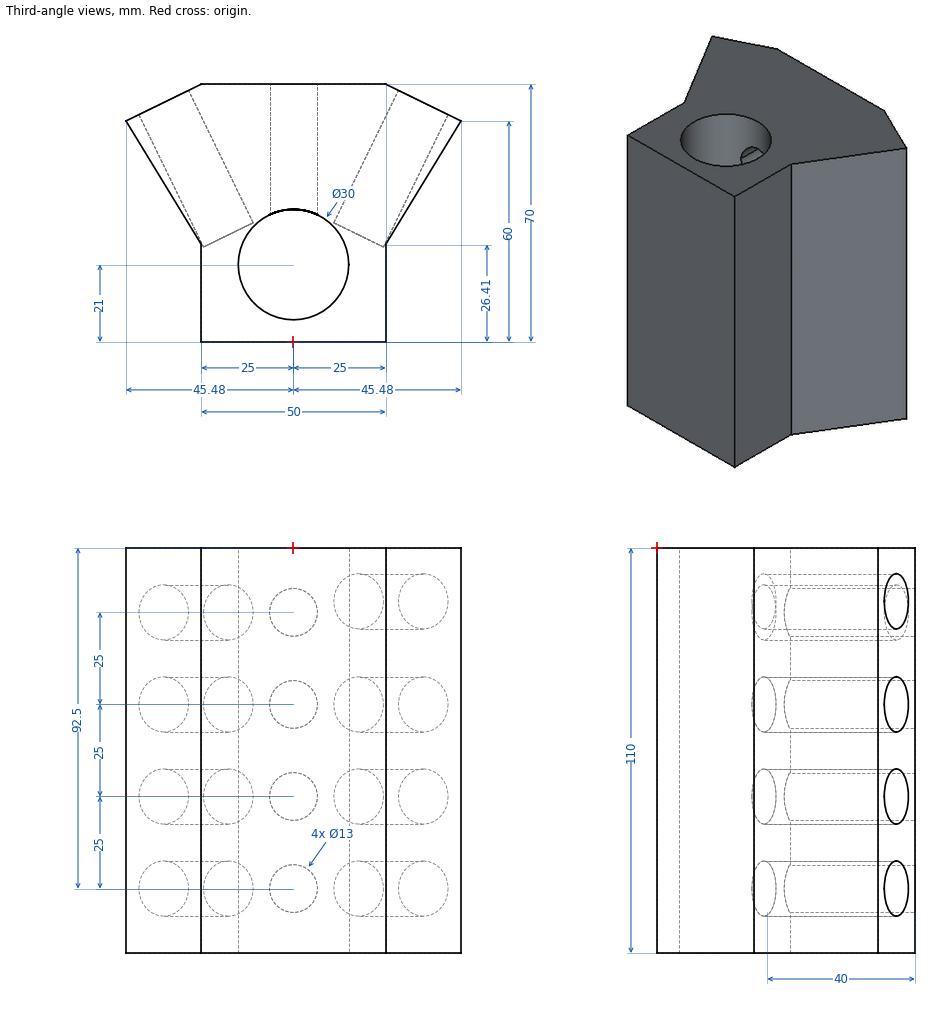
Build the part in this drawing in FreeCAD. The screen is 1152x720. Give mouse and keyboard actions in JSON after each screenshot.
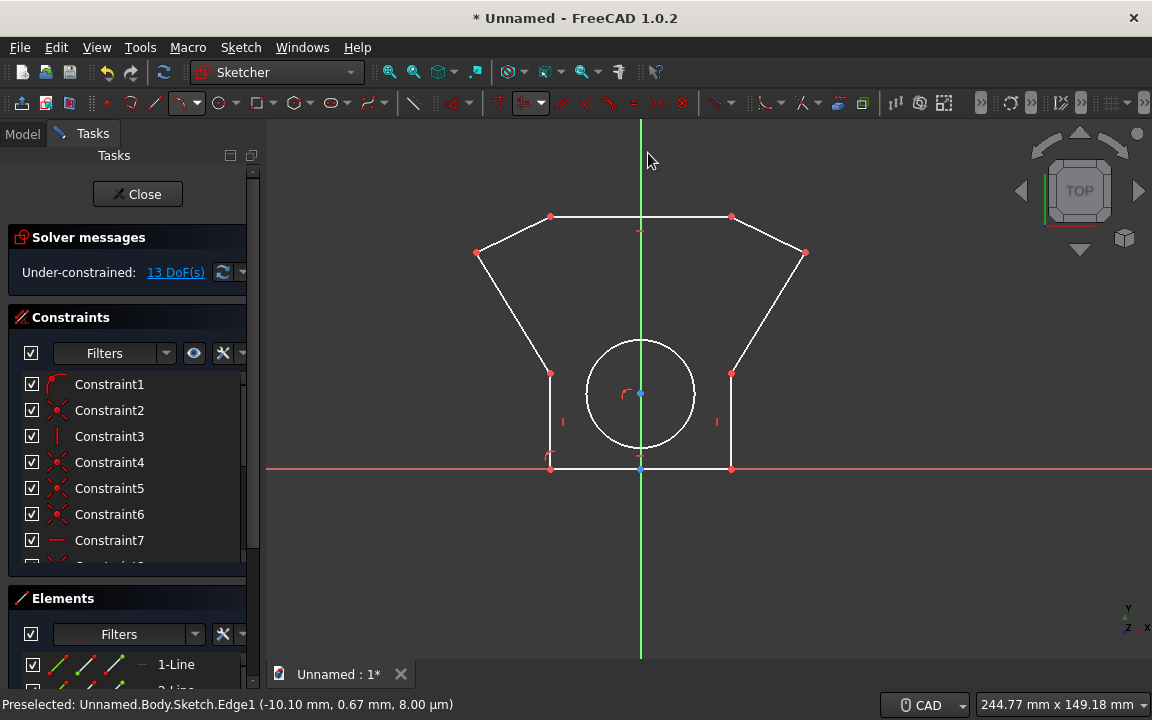
{"action": "left_click", "coordinate": [452, 104]}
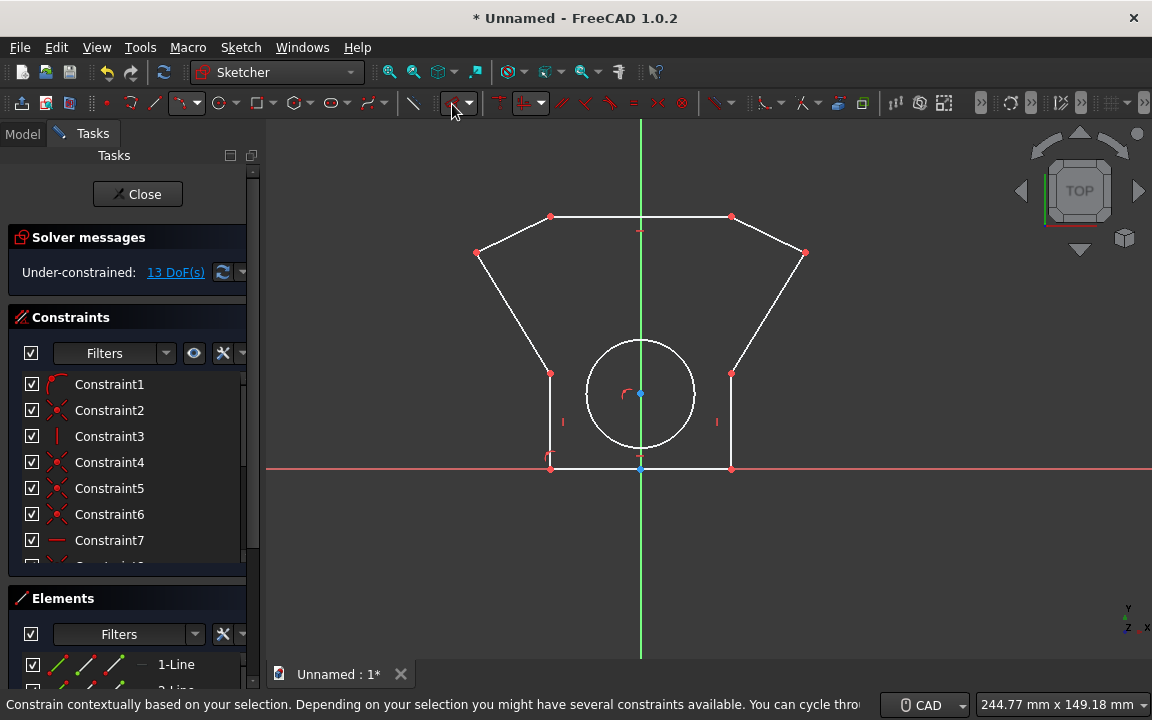
{"action": "left_click", "coordinate": [679, 356]}
{"action": "left_click", "coordinate": [702, 334]}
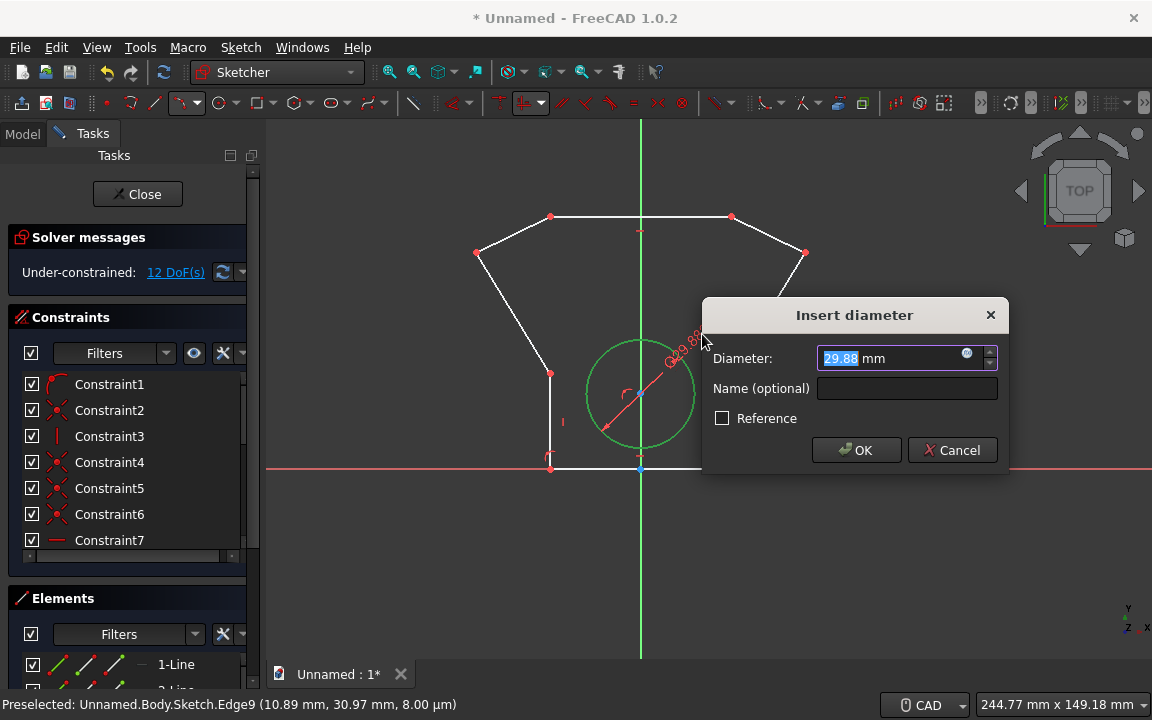
{"action": "type", "text": "30"}
{"action": "key", "text": "Return"}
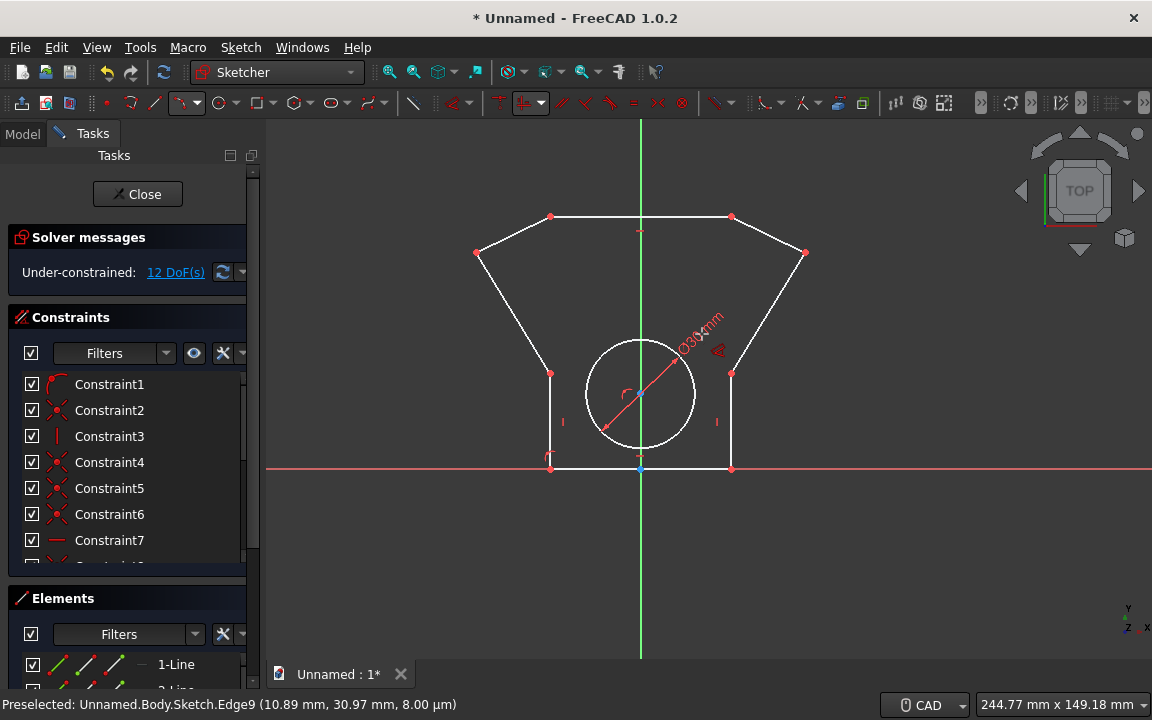
{"action": "left_click", "coordinate": [604, 469]}
{"action": "left_click", "coordinate": [599, 503]}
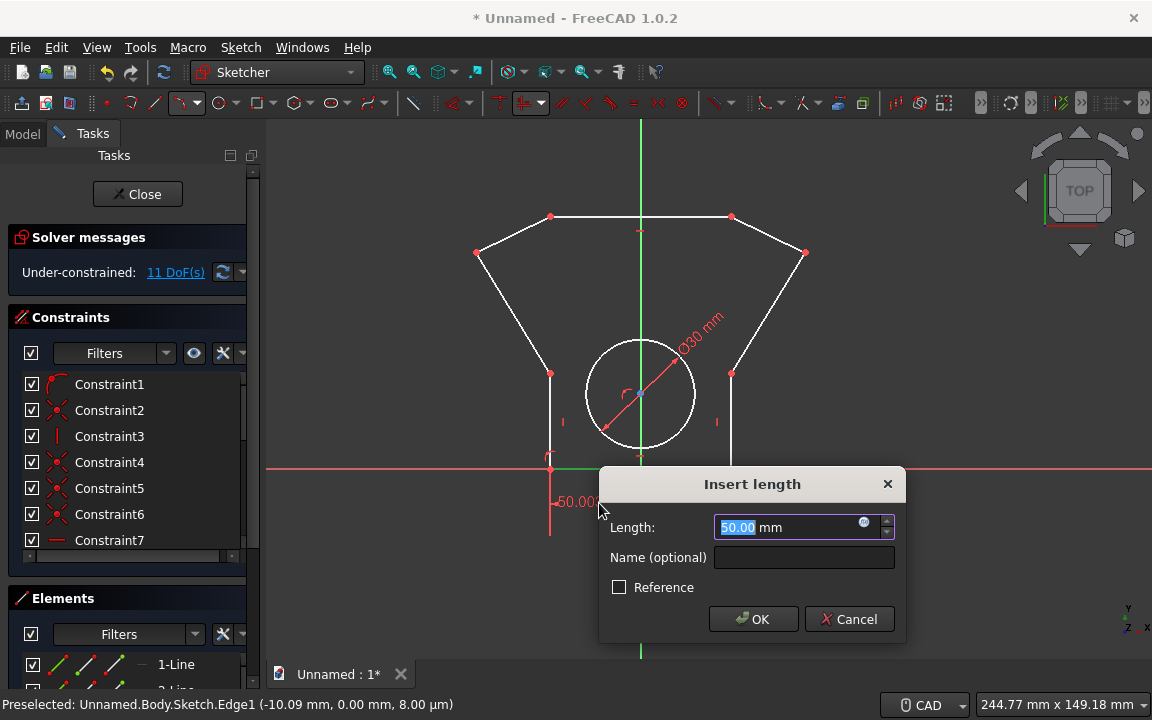
{"action": "type", "text": "50"}
{"action": "key", "text": "Return"}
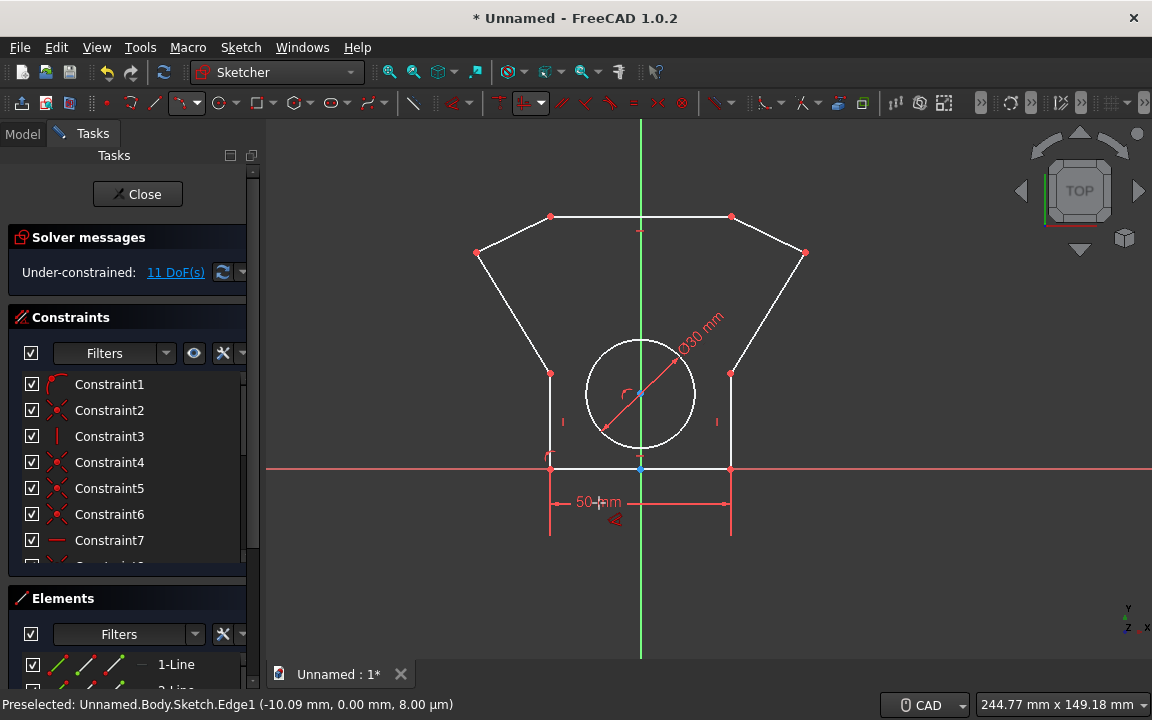
{"action": "left_click", "coordinate": [677, 217]}
{"action": "left_click", "coordinate": [599, 183]}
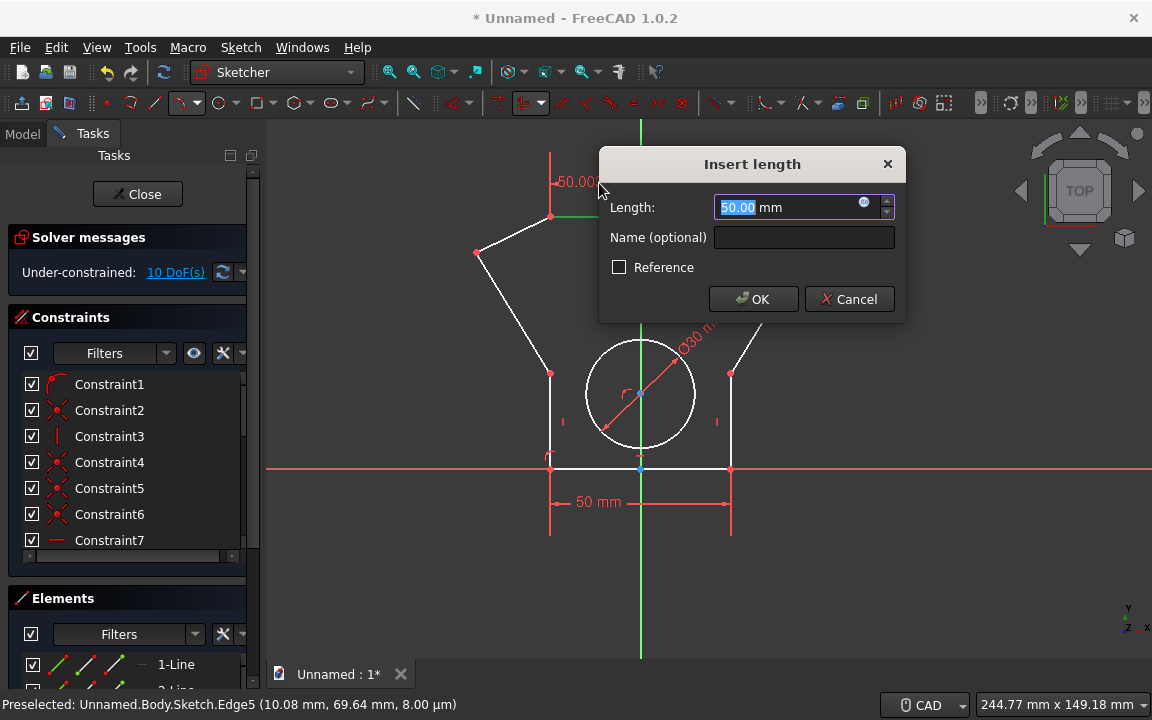
{"action": "type", "text": "50"}
{"action": "key", "text": "Return"}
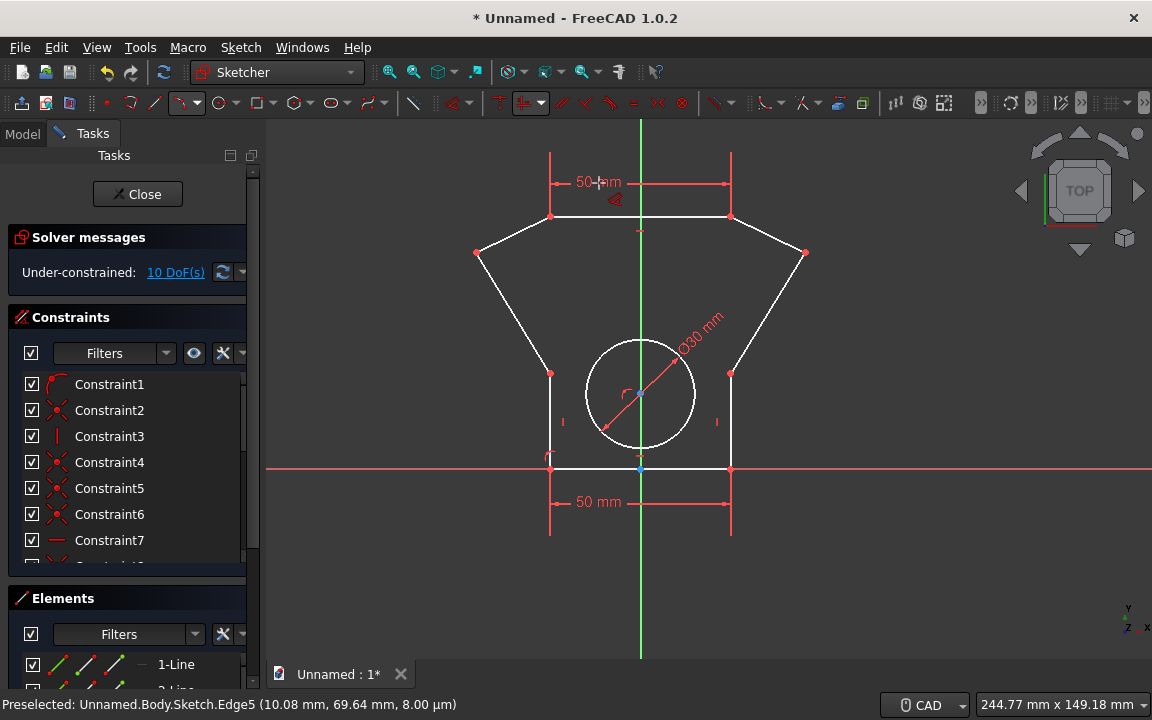
{"action": "left_click", "coordinate": [641, 394]}
{"action": "left_click", "coordinate": [675, 414]}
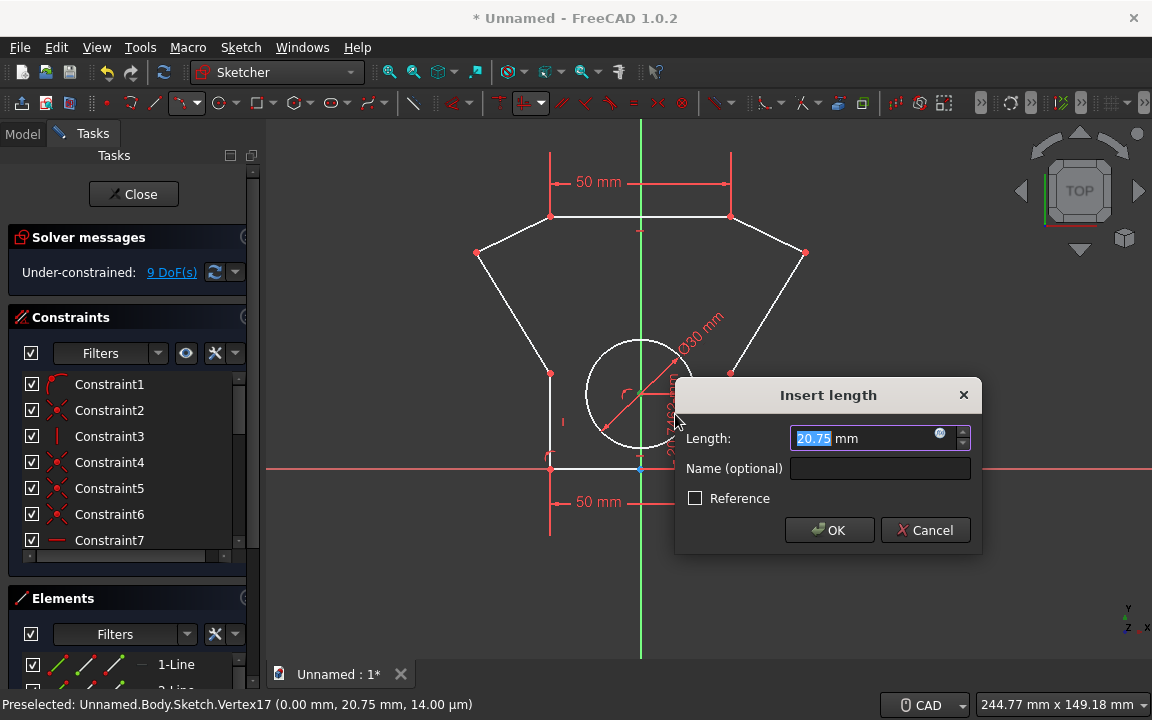
{"action": "type", "text": "21"}
{"action": "key", "text": "Return"}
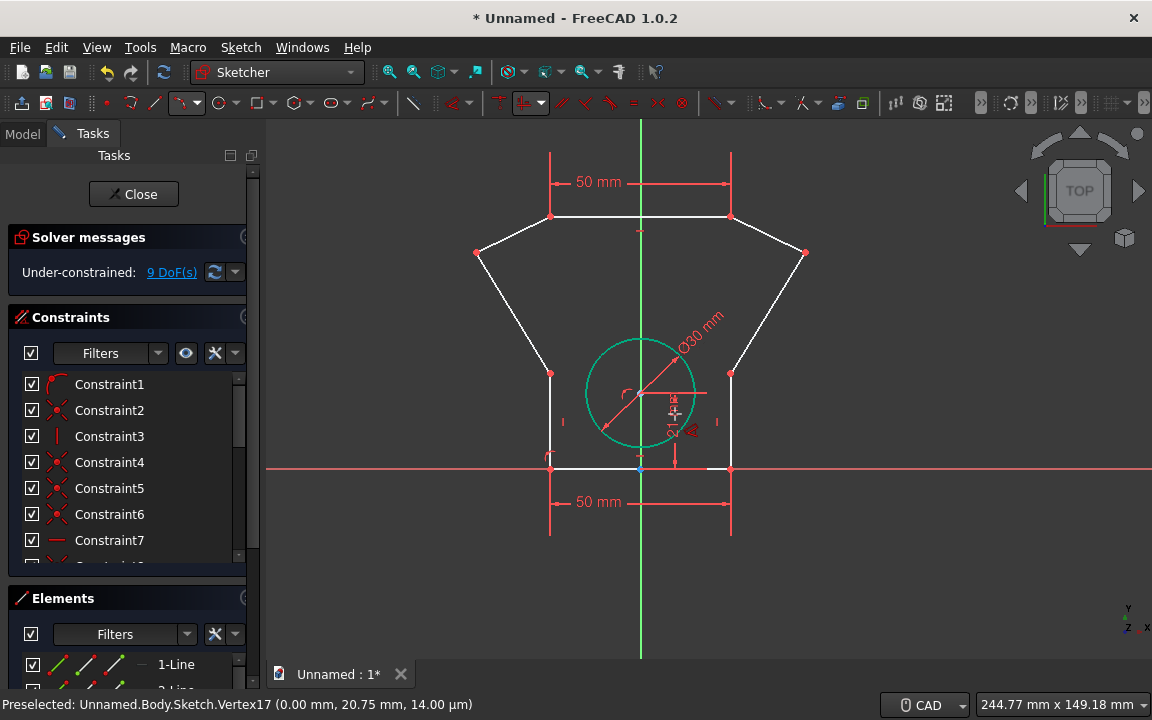
{"action": "left_click", "coordinate": [550, 469]}
{"action": "left_click", "coordinate": [574, 435]}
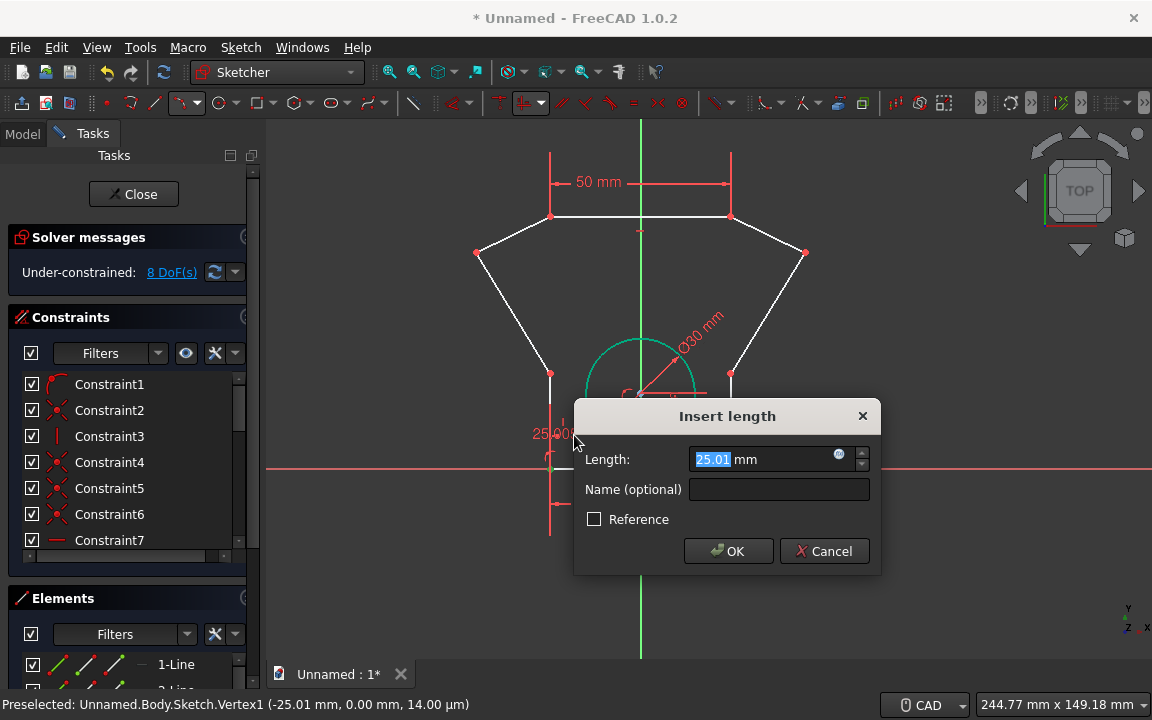
{"action": "type", "text": "25"}
{"action": "key", "text": "Return"}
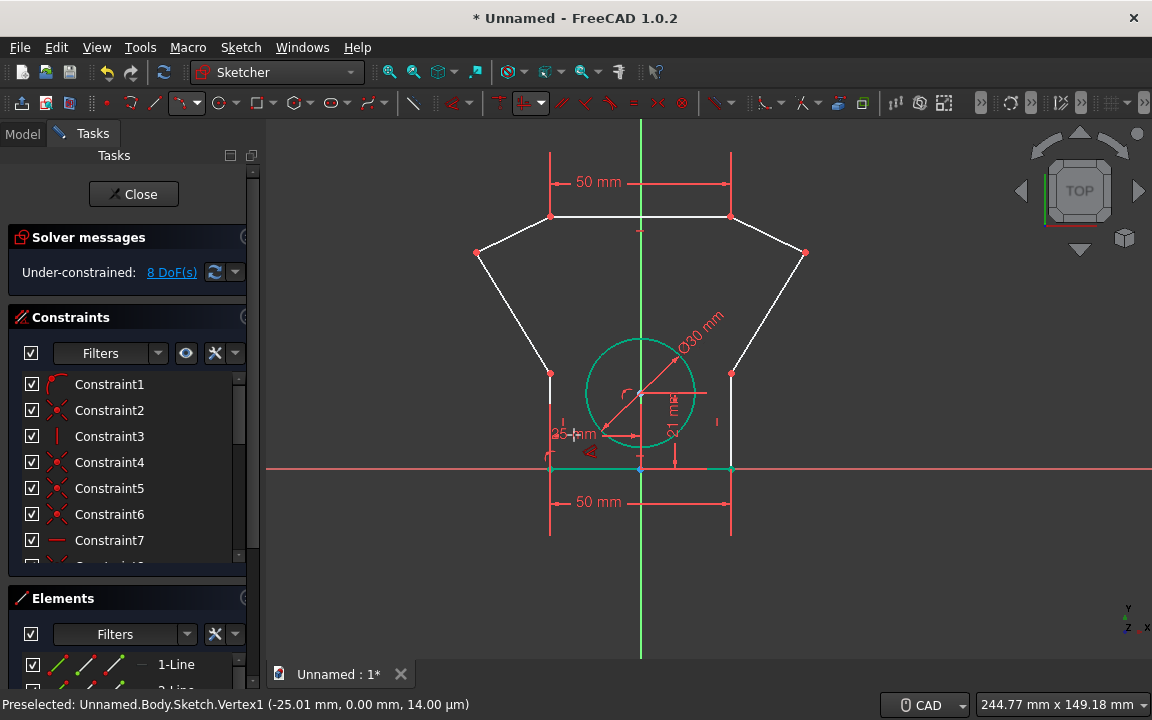
{"action": "left_click", "coordinate": [805, 253]}
{"action": "left_click", "coordinate": [839, 361]}